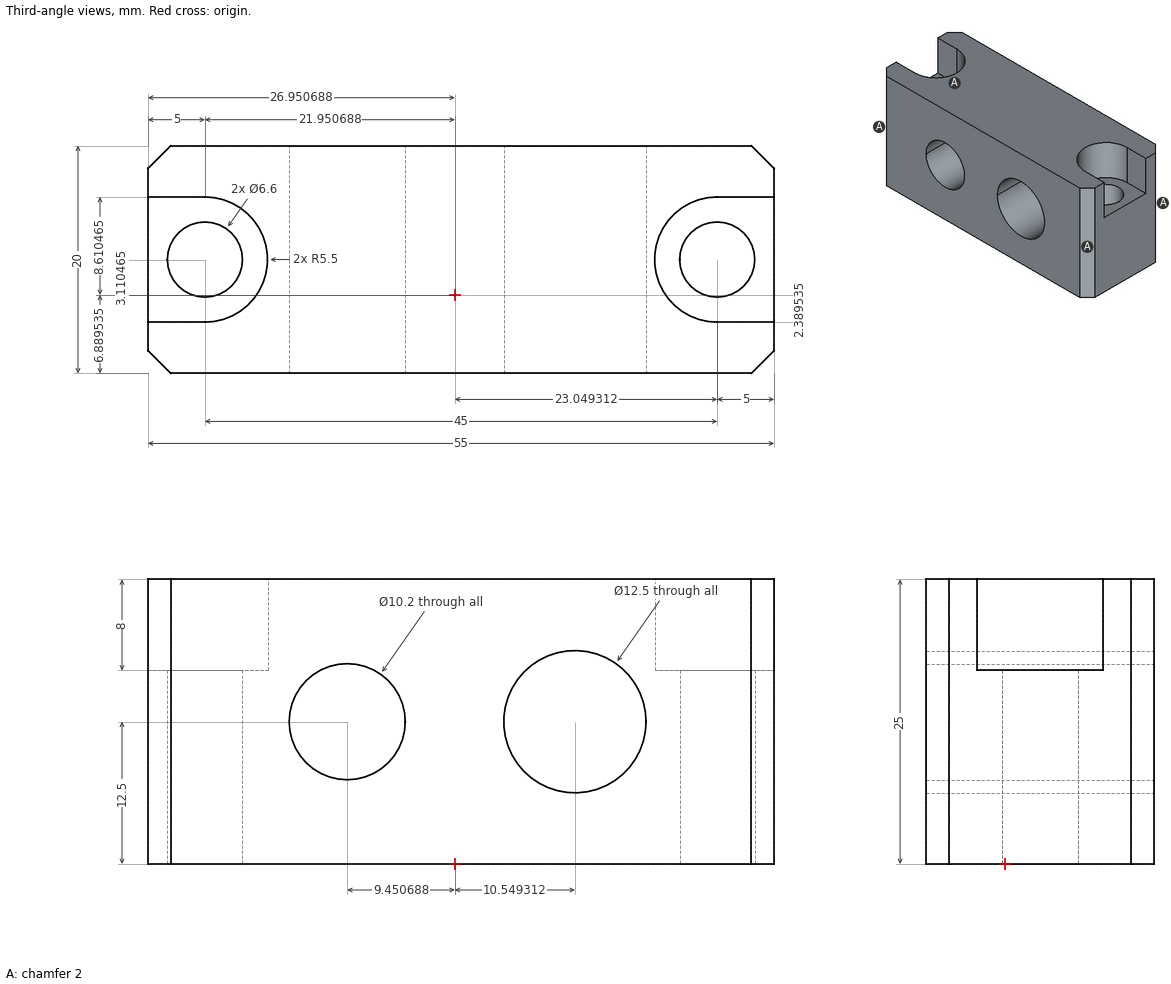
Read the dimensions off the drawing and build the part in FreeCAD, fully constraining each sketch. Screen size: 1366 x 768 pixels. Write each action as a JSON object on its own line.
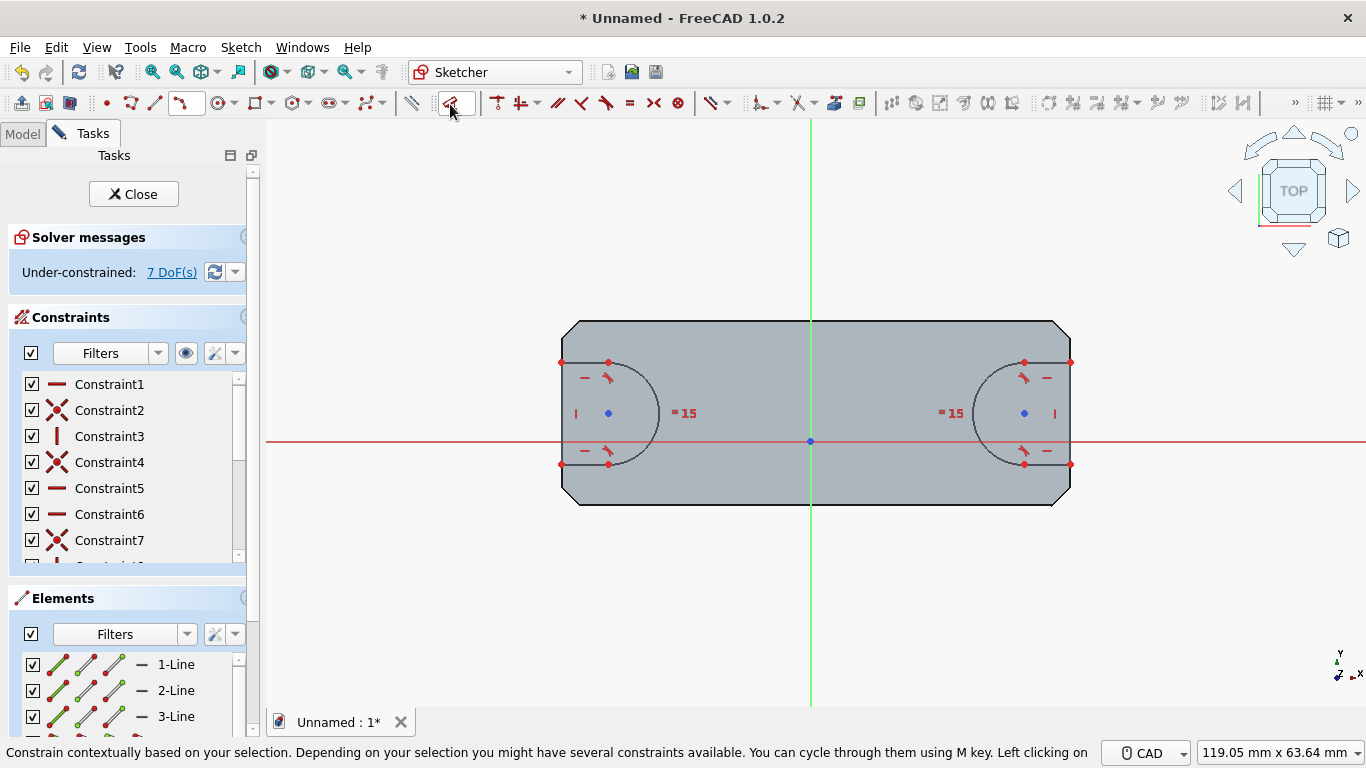
{"action": "left_click", "coordinate": [649, 444]}
{"action": "left_click", "coordinate": [675, 463]}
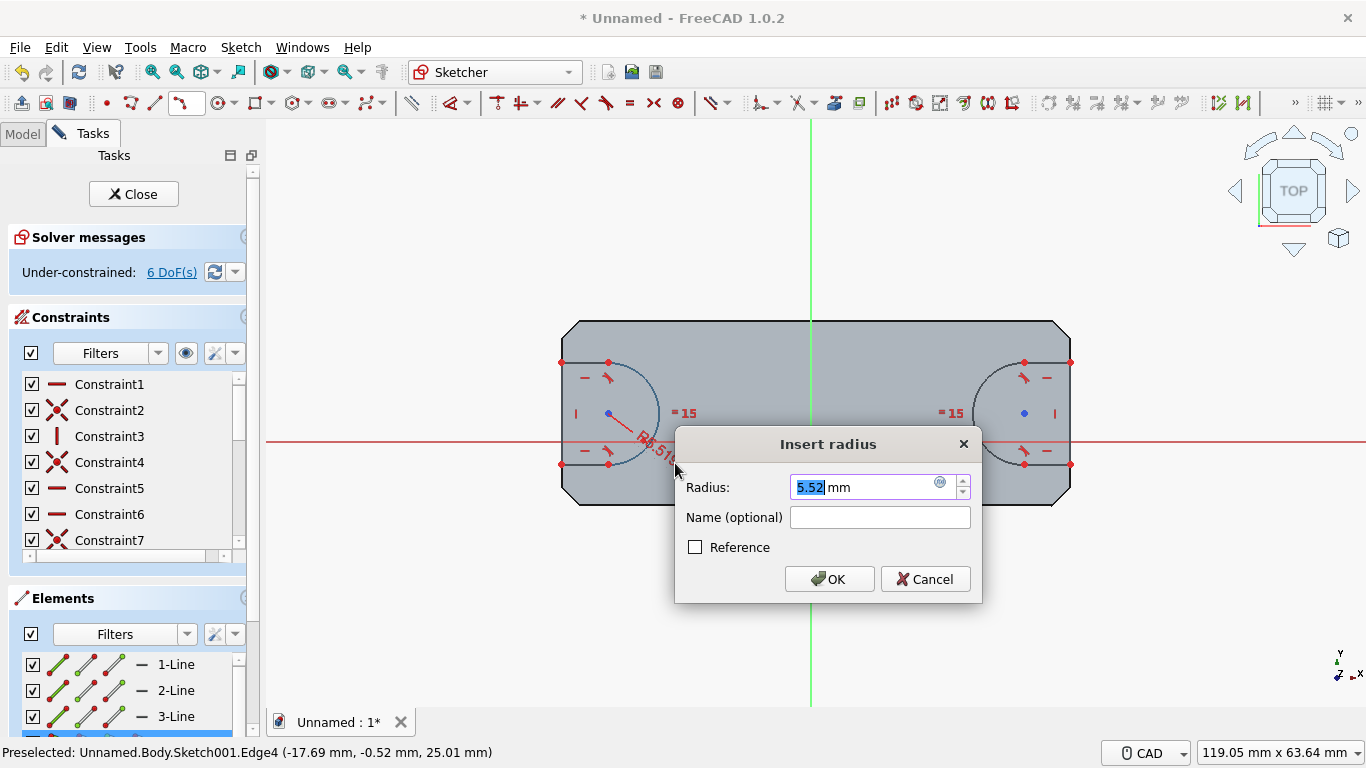
{"action": "type", "text": "5.5"}
{"action": "key", "text": "Return"}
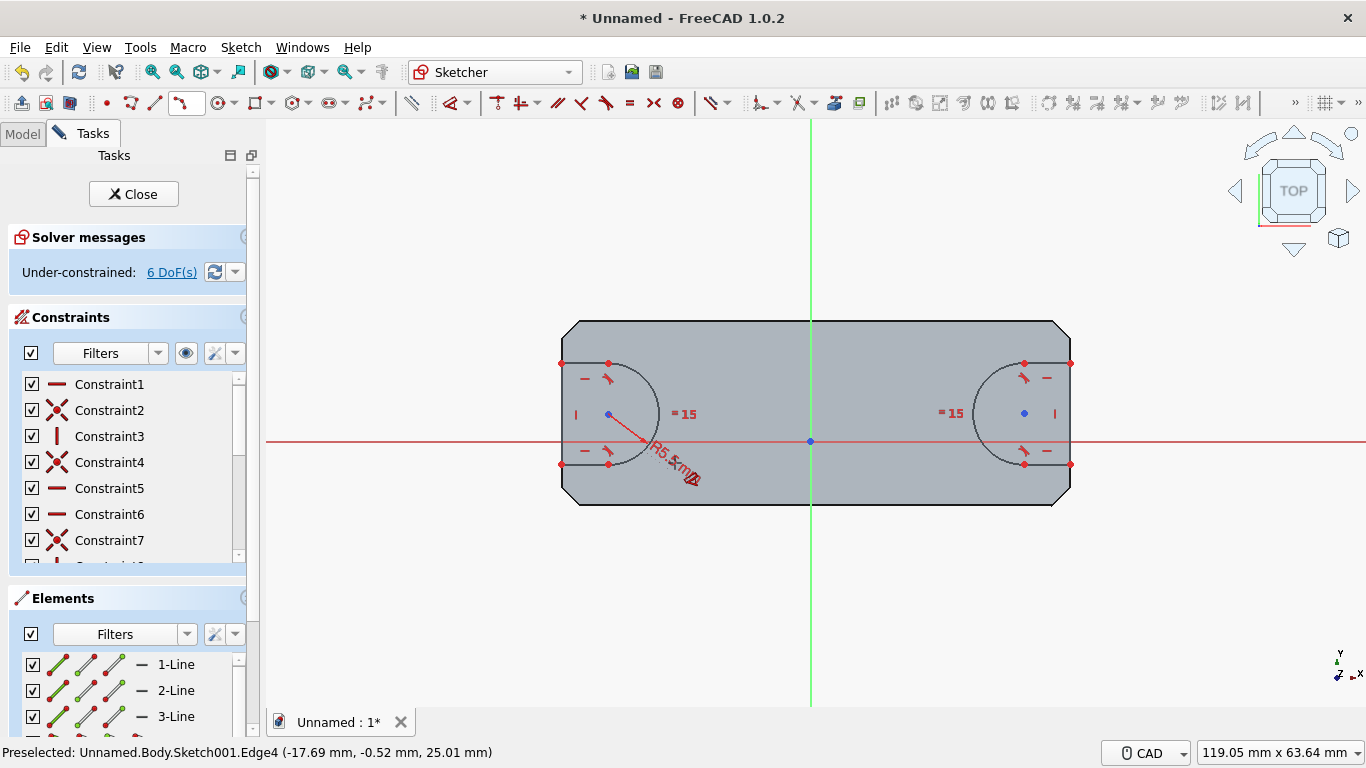
{"action": "left_click", "coordinate": [594, 363]}
{"action": "left_click", "coordinate": [585, 329]}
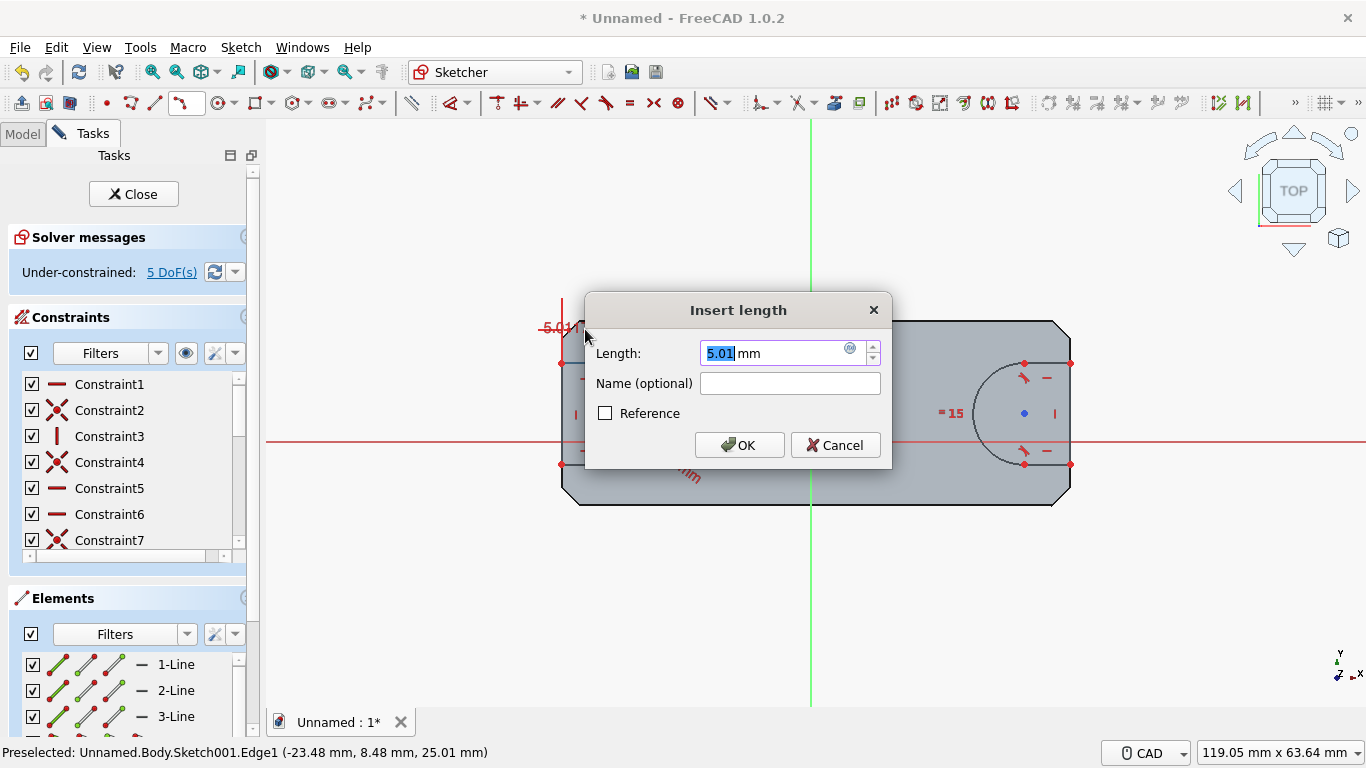
{"action": "type", "text": "5"}
{"action": "key", "text": "Return"}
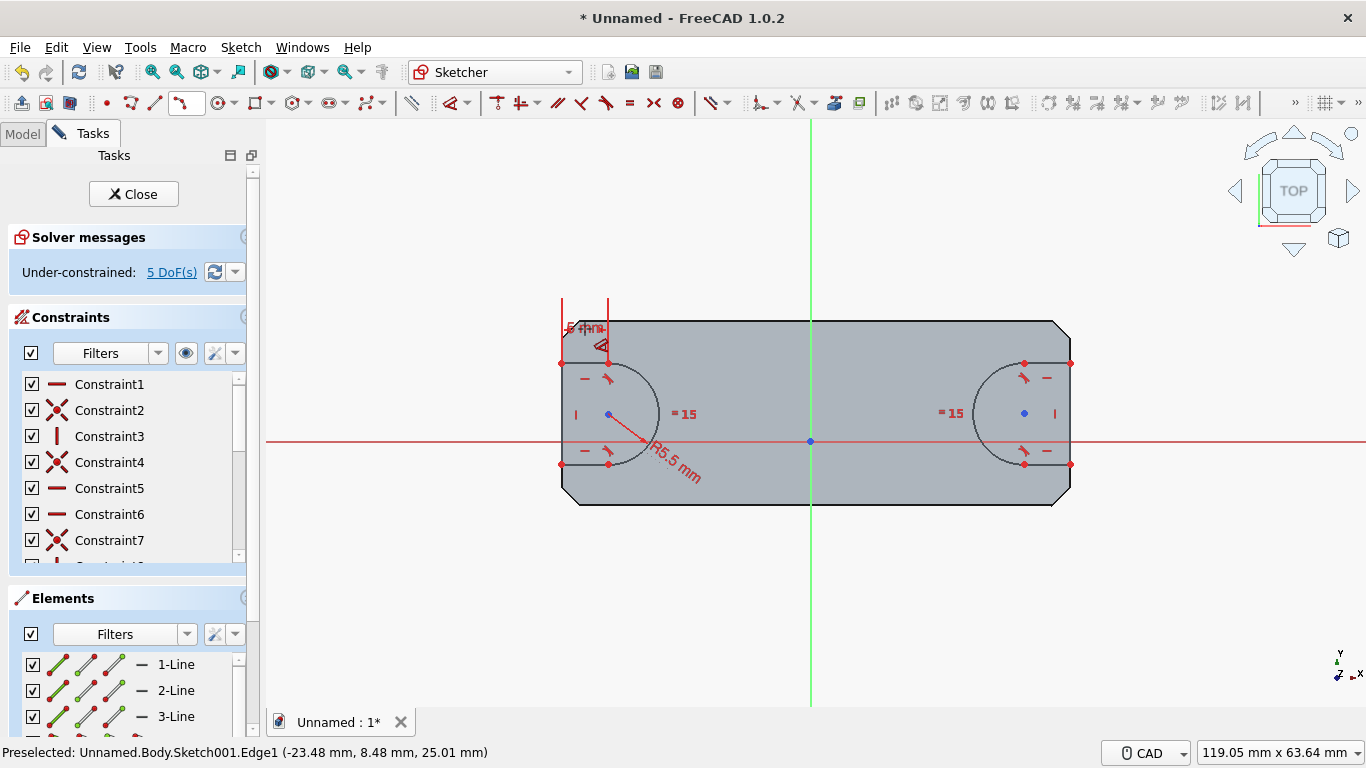
{"action": "left_click", "coordinate": [1038, 465]}
{"action": "left_click", "coordinate": [1047, 499]}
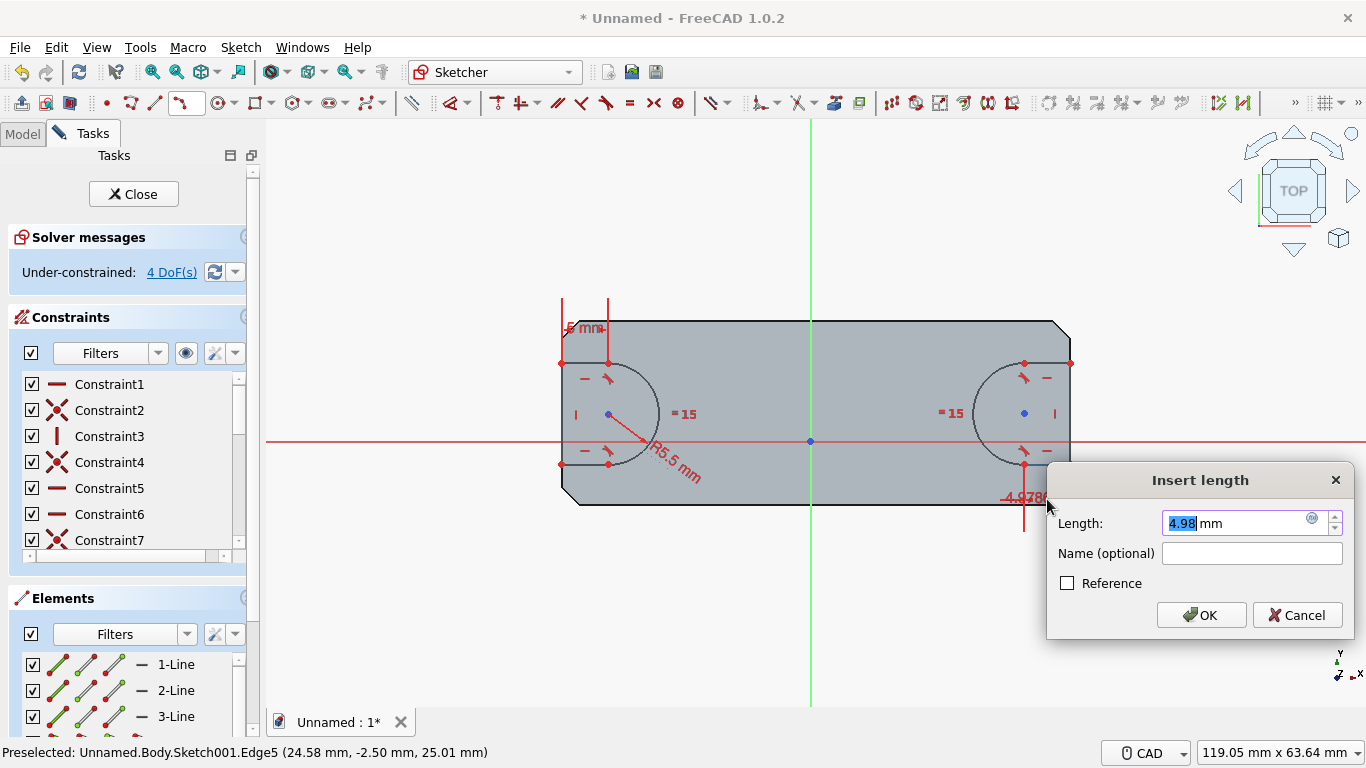
{"action": "type", "text": "5"}
{"action": "key", "text": "Return"}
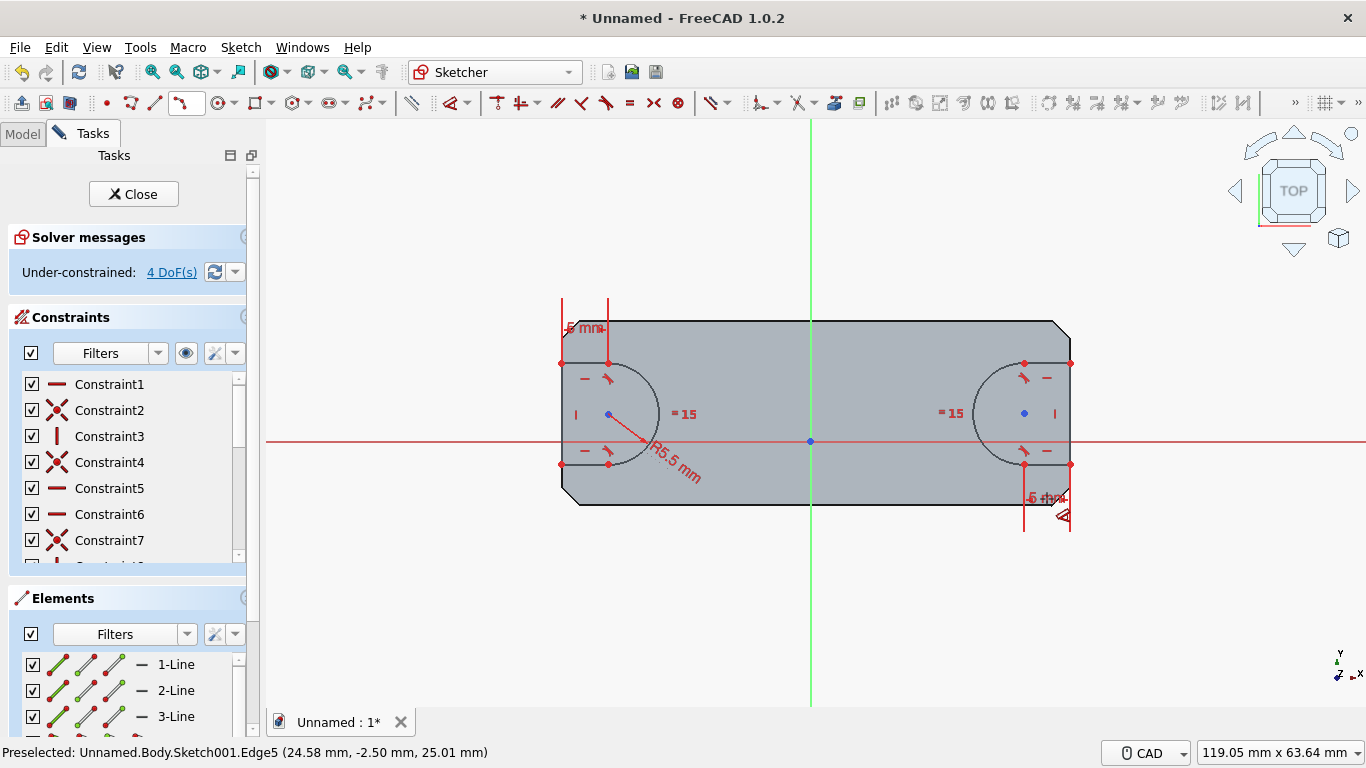
{"action": "left_click", "coordinate": [608, 363]}
{"action": "left_click", "coordinate": [845, 403]}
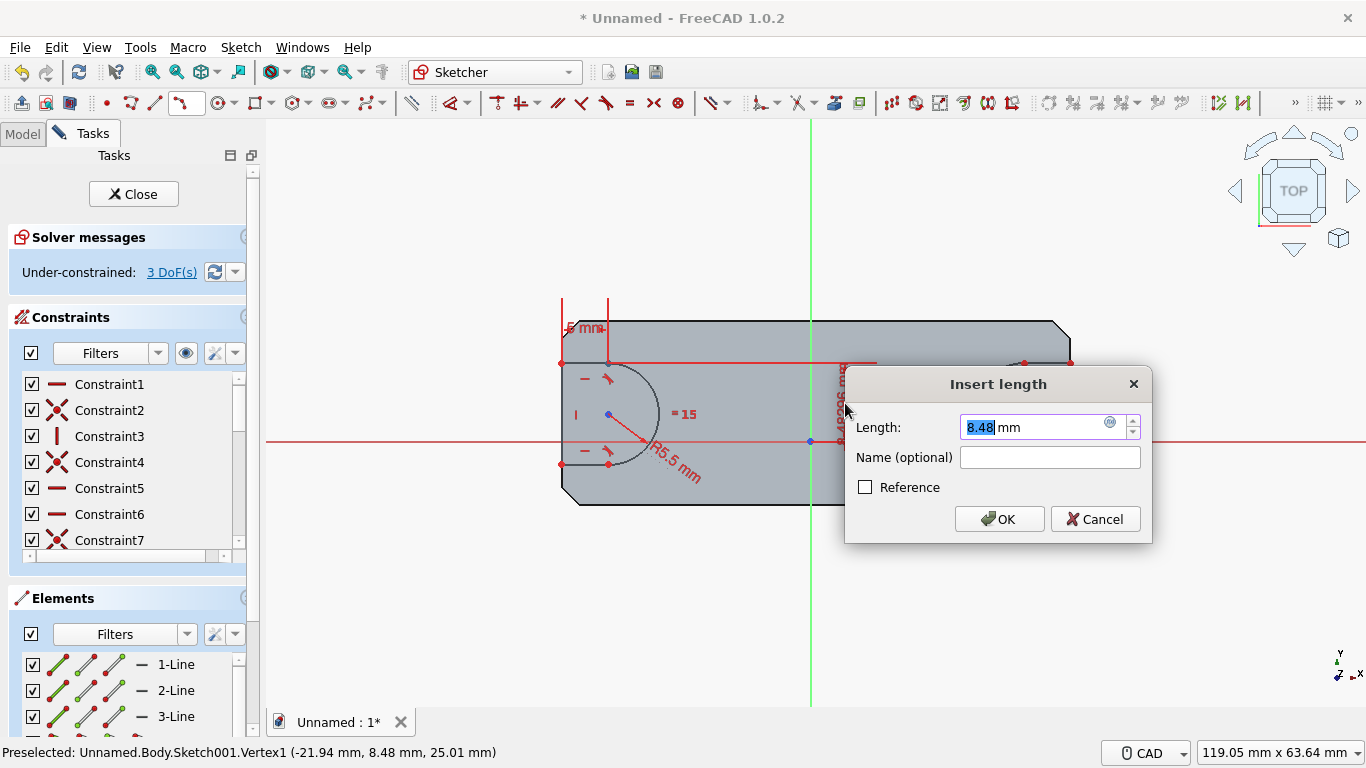
{"action": "type", "text": "8.610465"}
{"action": "key", "text": "Return"}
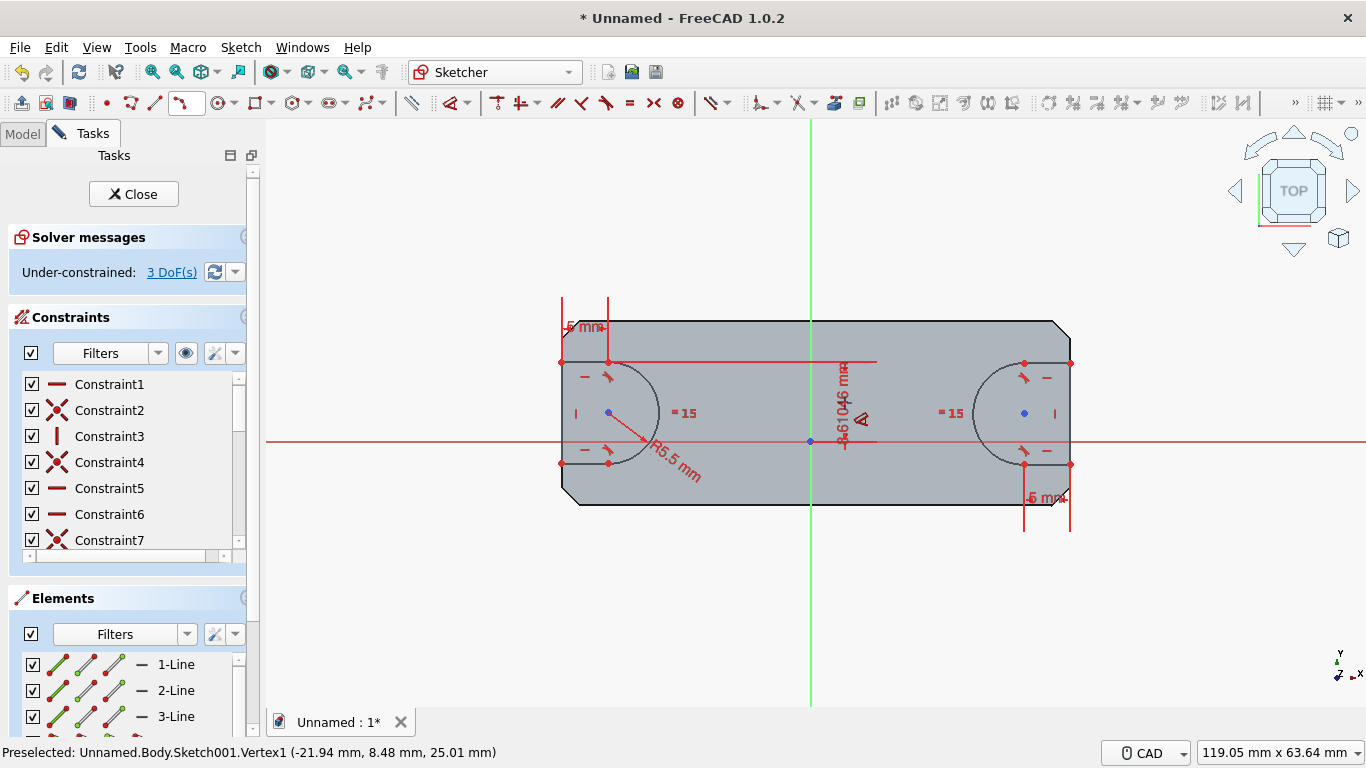
{"action": "scroll", "coordinate": [1024, 465], "scroll_direction": "up", "scroll_amount": 3}